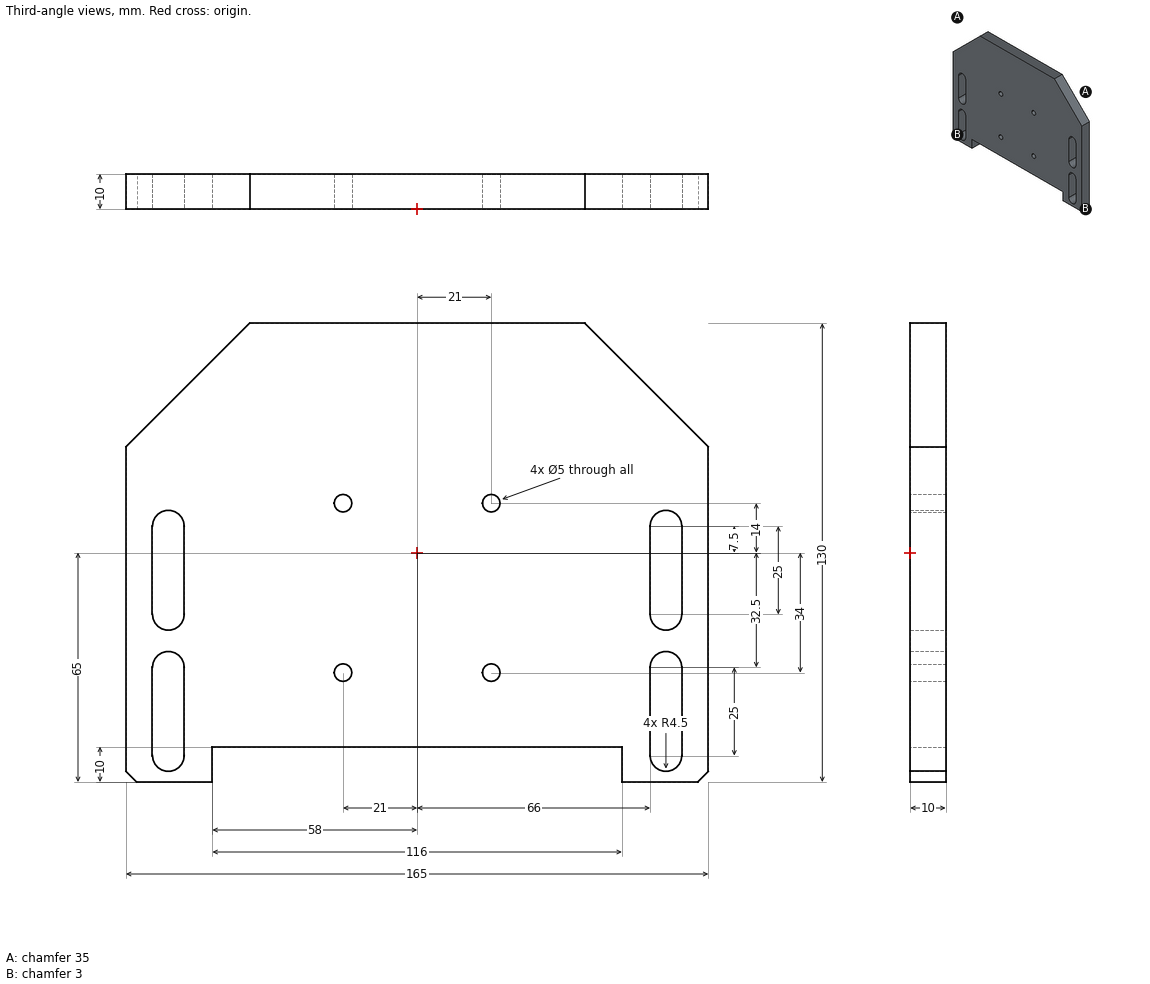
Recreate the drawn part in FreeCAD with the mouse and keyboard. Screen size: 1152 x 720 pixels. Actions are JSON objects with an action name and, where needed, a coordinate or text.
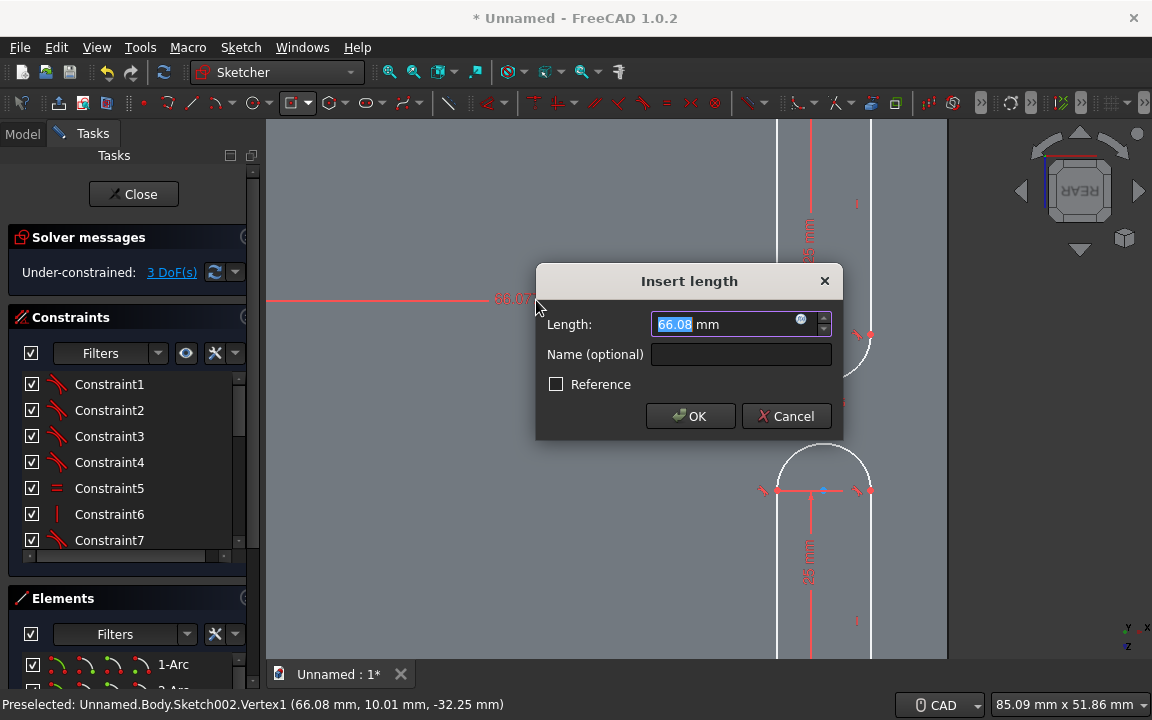
{"action": "type", "text": "66"}
{"action": "key", "text": "Return"}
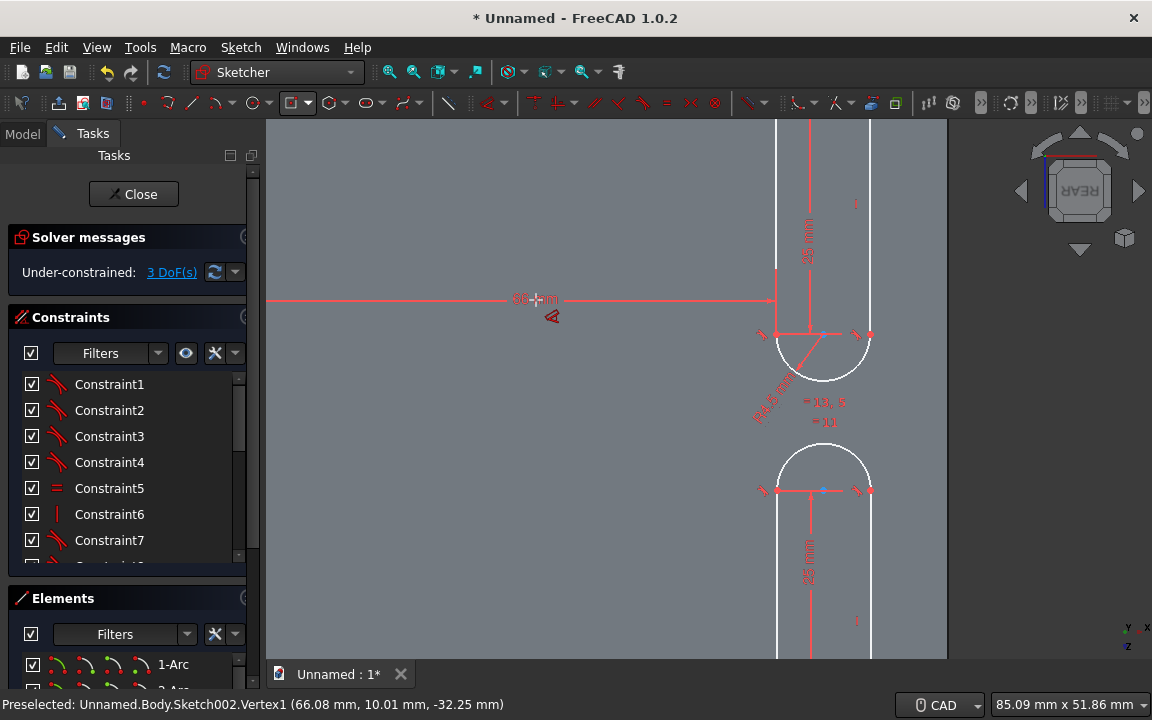
{"action": "scroll", "coordinate": [772, 372], "scroll_direction": "down", "scroll_amount": 4}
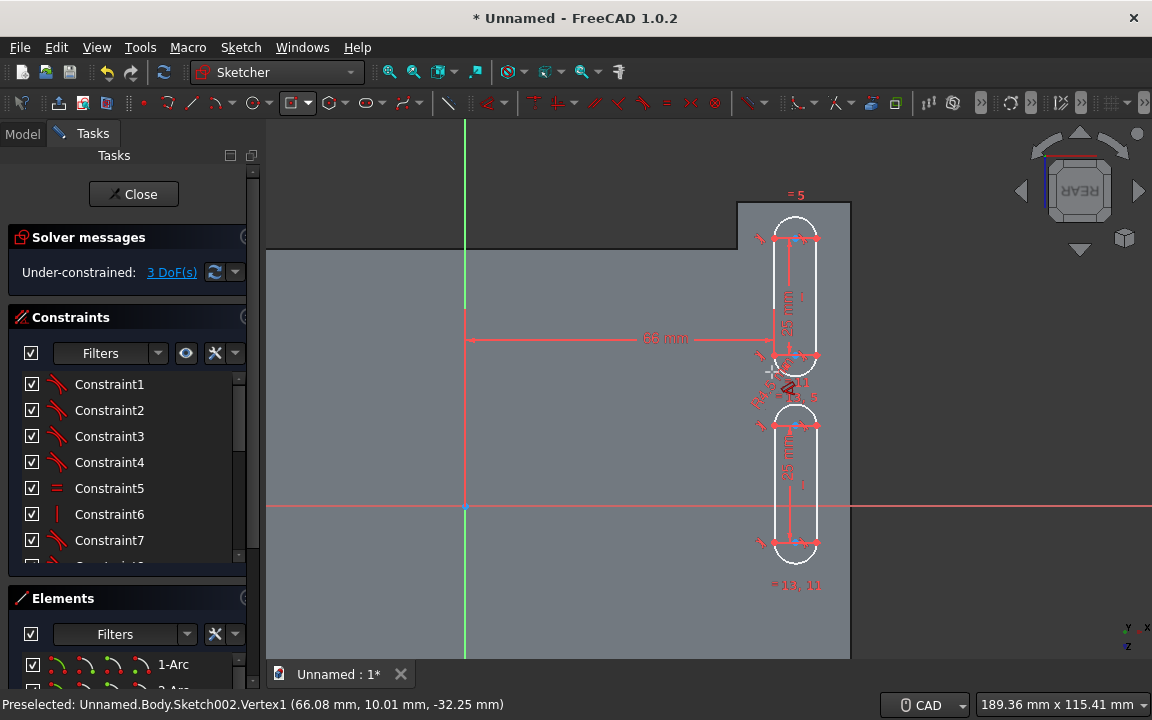
{"action": "left_click", "coordinate": [775, 543]}
{"action": "left_click", "coordinate": [620, 577]}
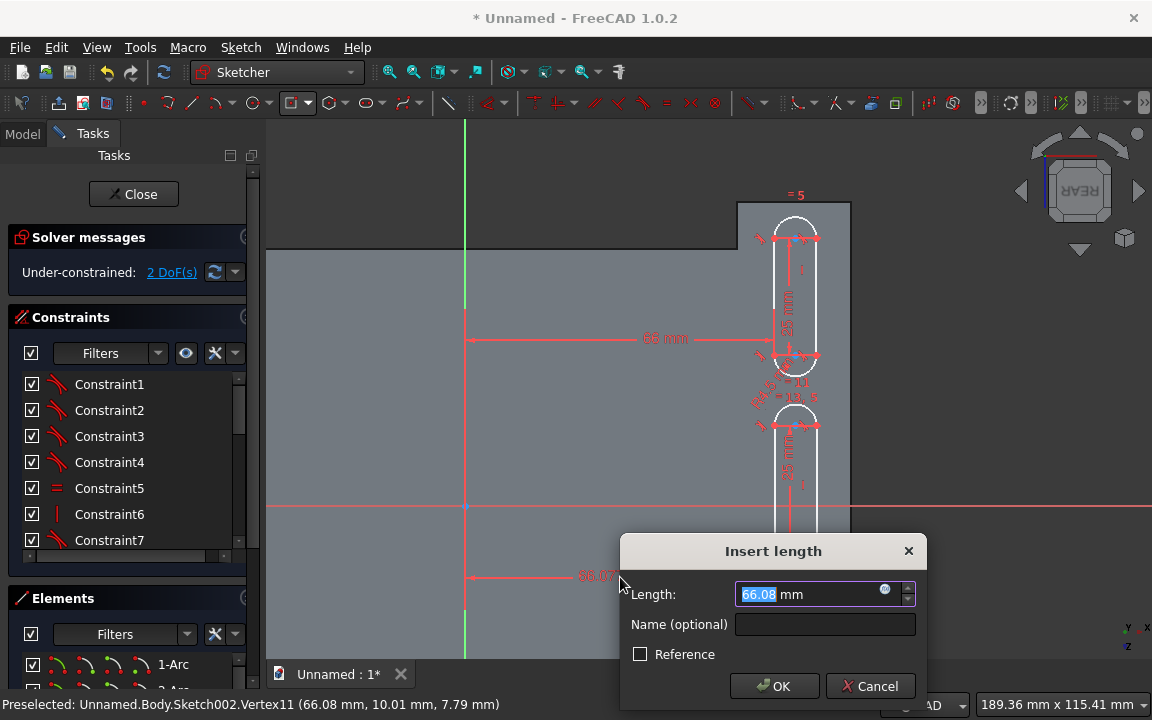
{"action": "type", "text": "66"}
{"action": "key", "text": "Return"}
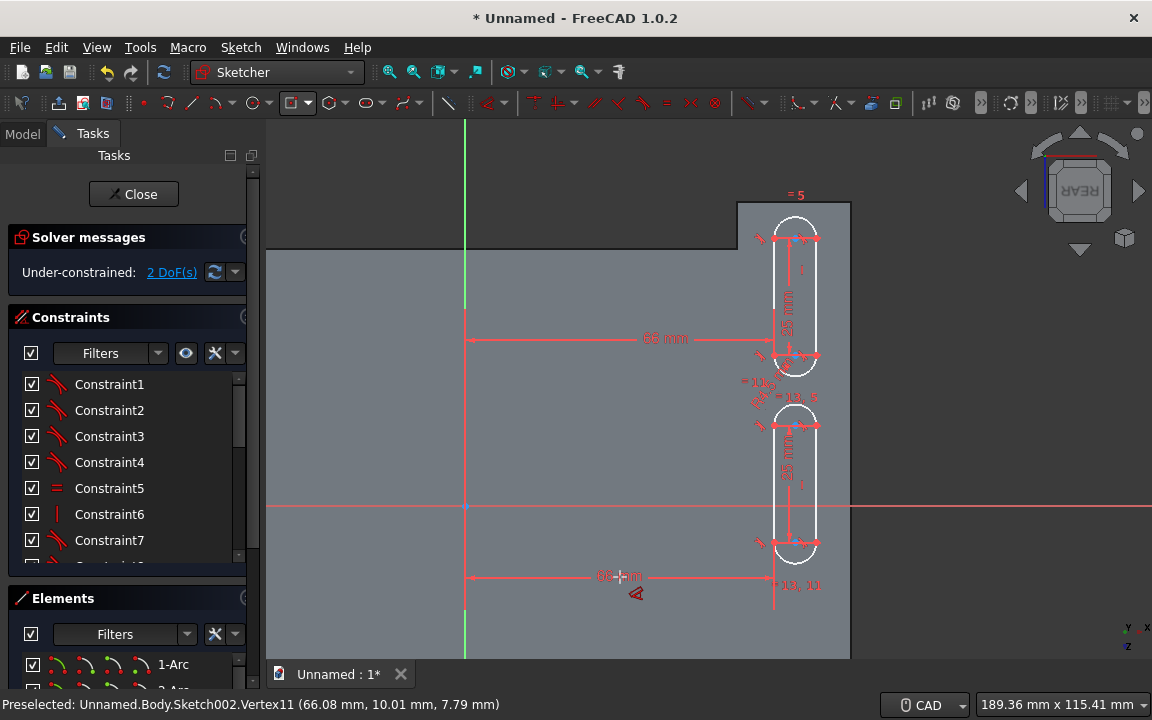
{"action": "left_click", "coordinate": [774, 543]}
{"action": "left_click", "coordinate": [431, 524]}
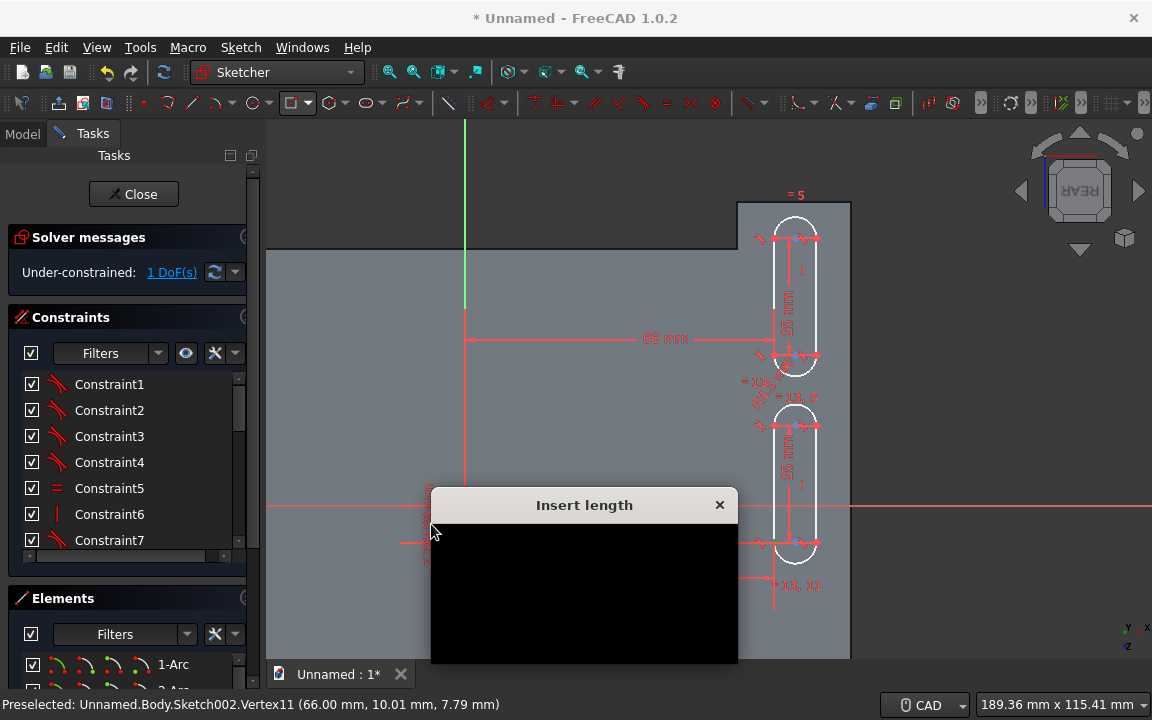
{"action": "type", "text": "7.5"}
{"action": "key", "text": "Return"}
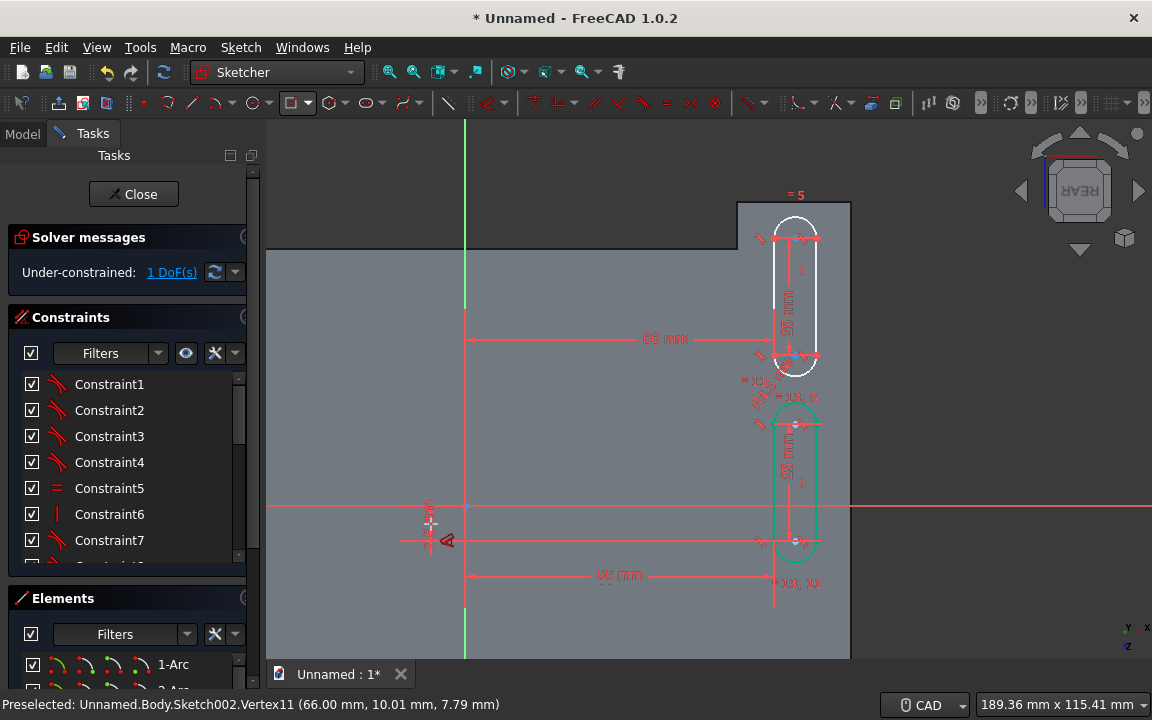
{"action": "left_click", "coordinate": [774, 355]}
{"action": "left_click", "coordinate": [431, 431]}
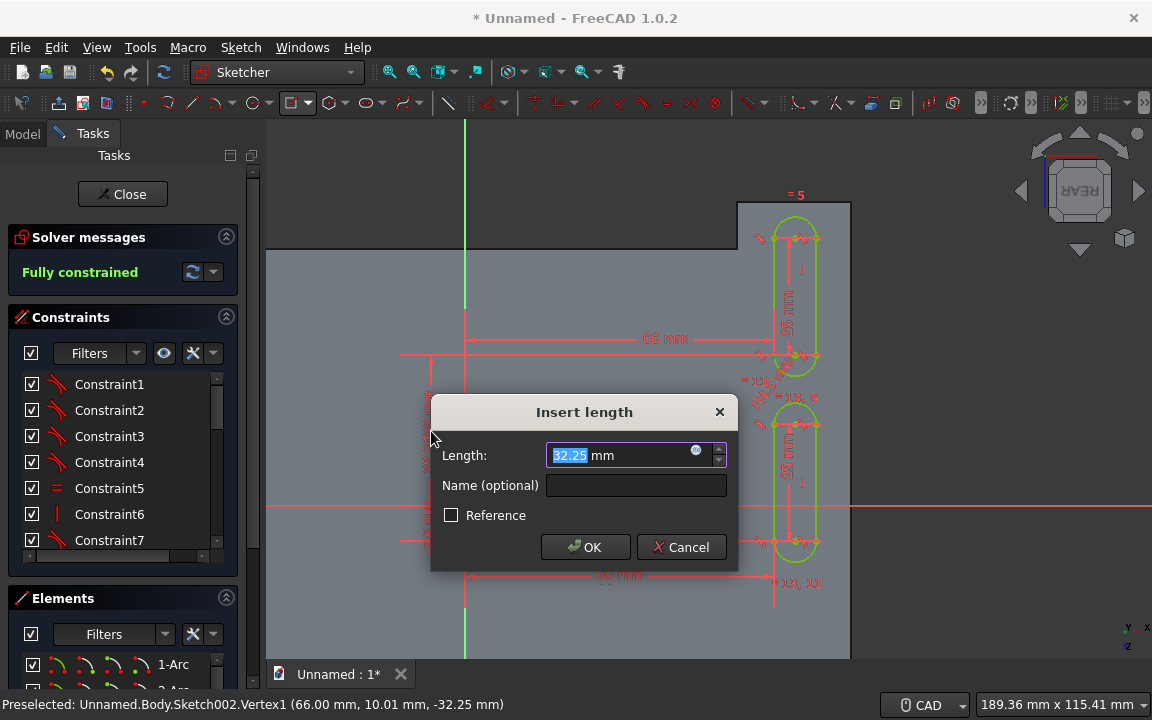
{"action": "type", "text": "32.5"}
{"action": "key", "text": "Return"}
{"action": "key", "text": "Escape"}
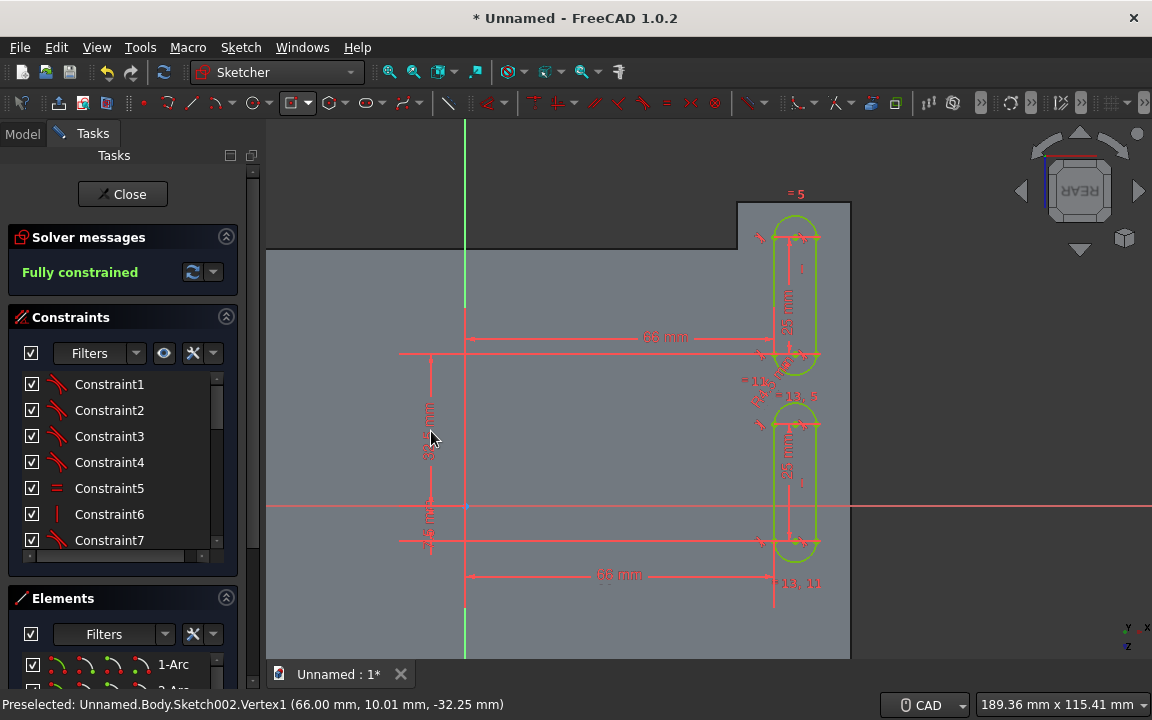
{"action": "left_click", "coordinate": [123, 194]}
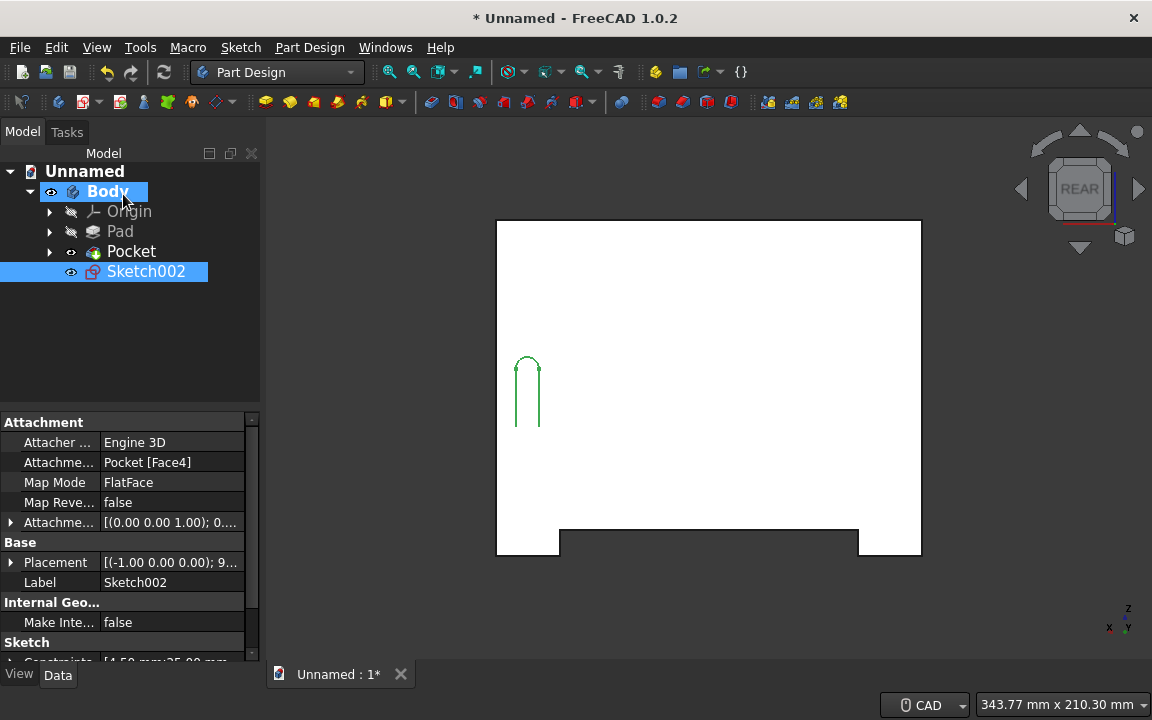
{"action": "left_click", "coordinate": [432, 102]}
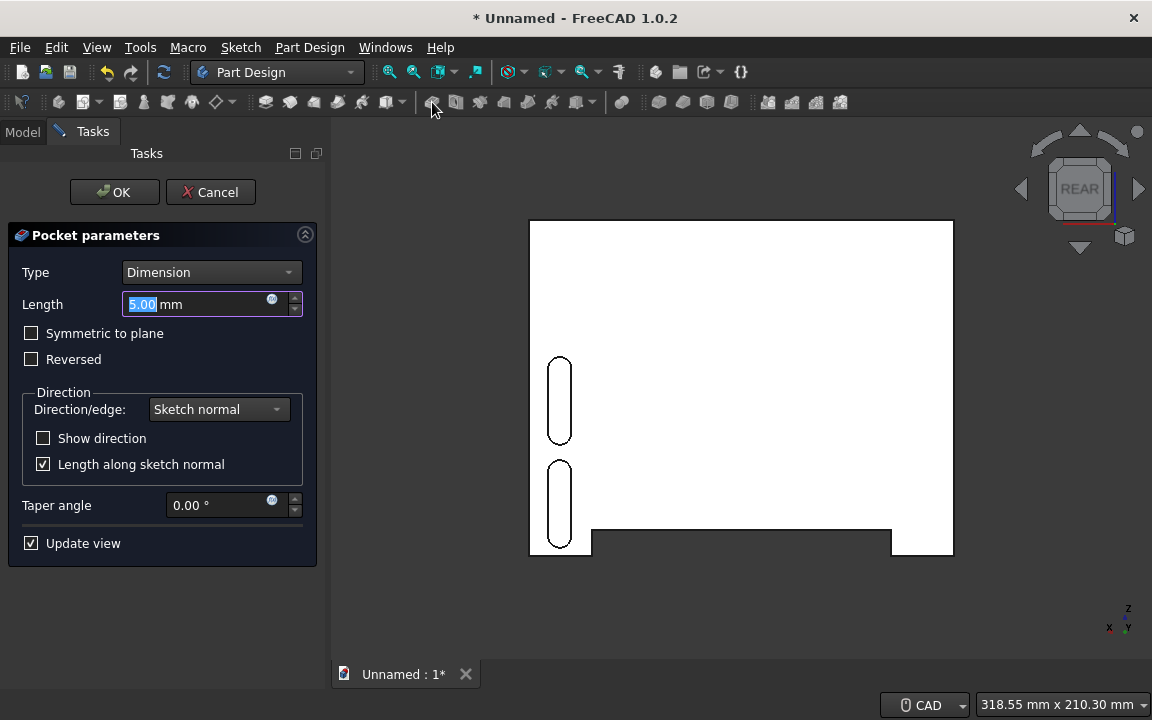
{"action": "left_click", "coordinate": [212, 272]}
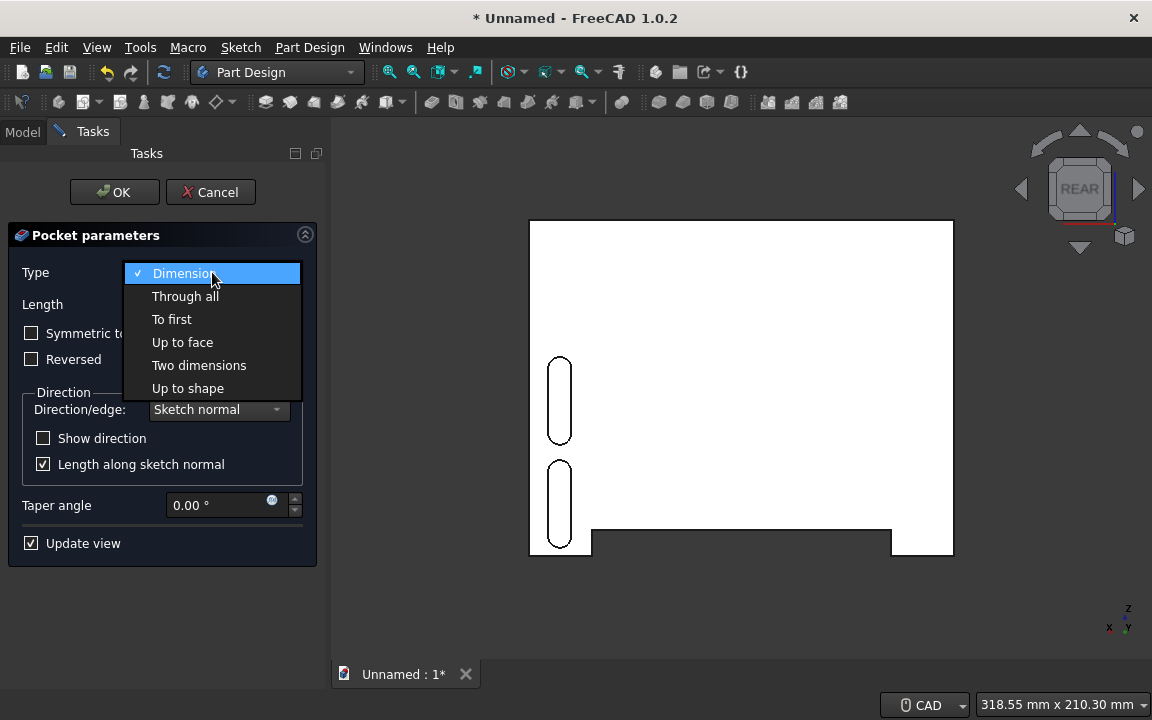
{"action": "left_click", "coordinate": [212, 296]}